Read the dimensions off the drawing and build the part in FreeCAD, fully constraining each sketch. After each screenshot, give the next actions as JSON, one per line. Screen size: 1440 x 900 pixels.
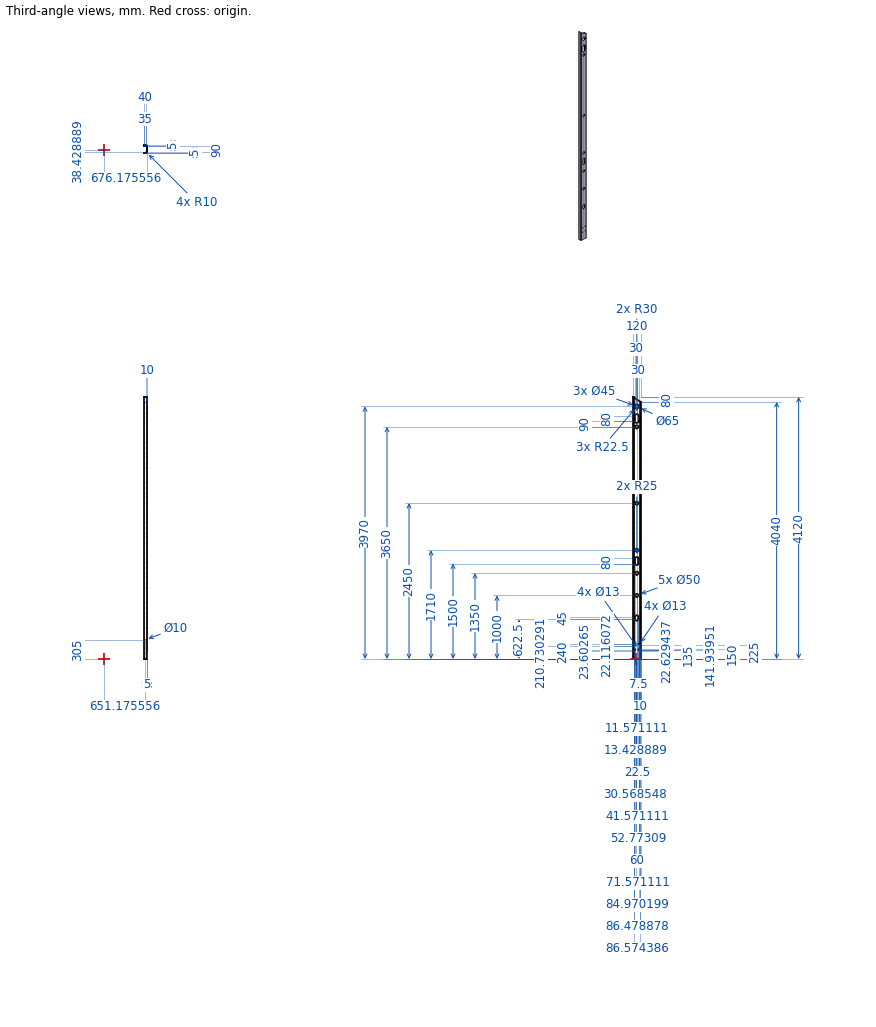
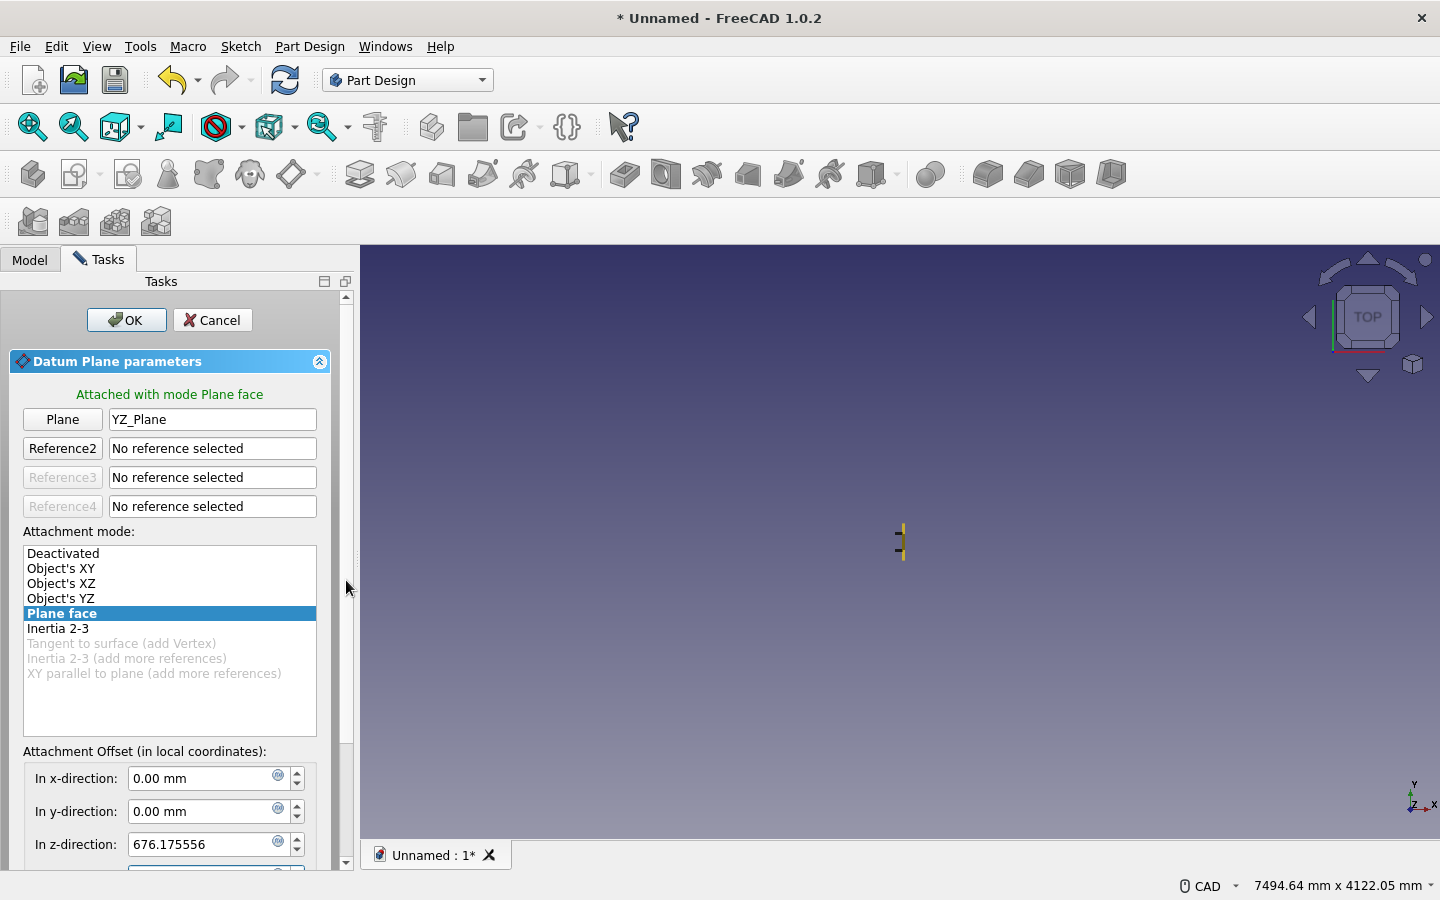
{"action": "left_click", "coordinate": [127, 320]}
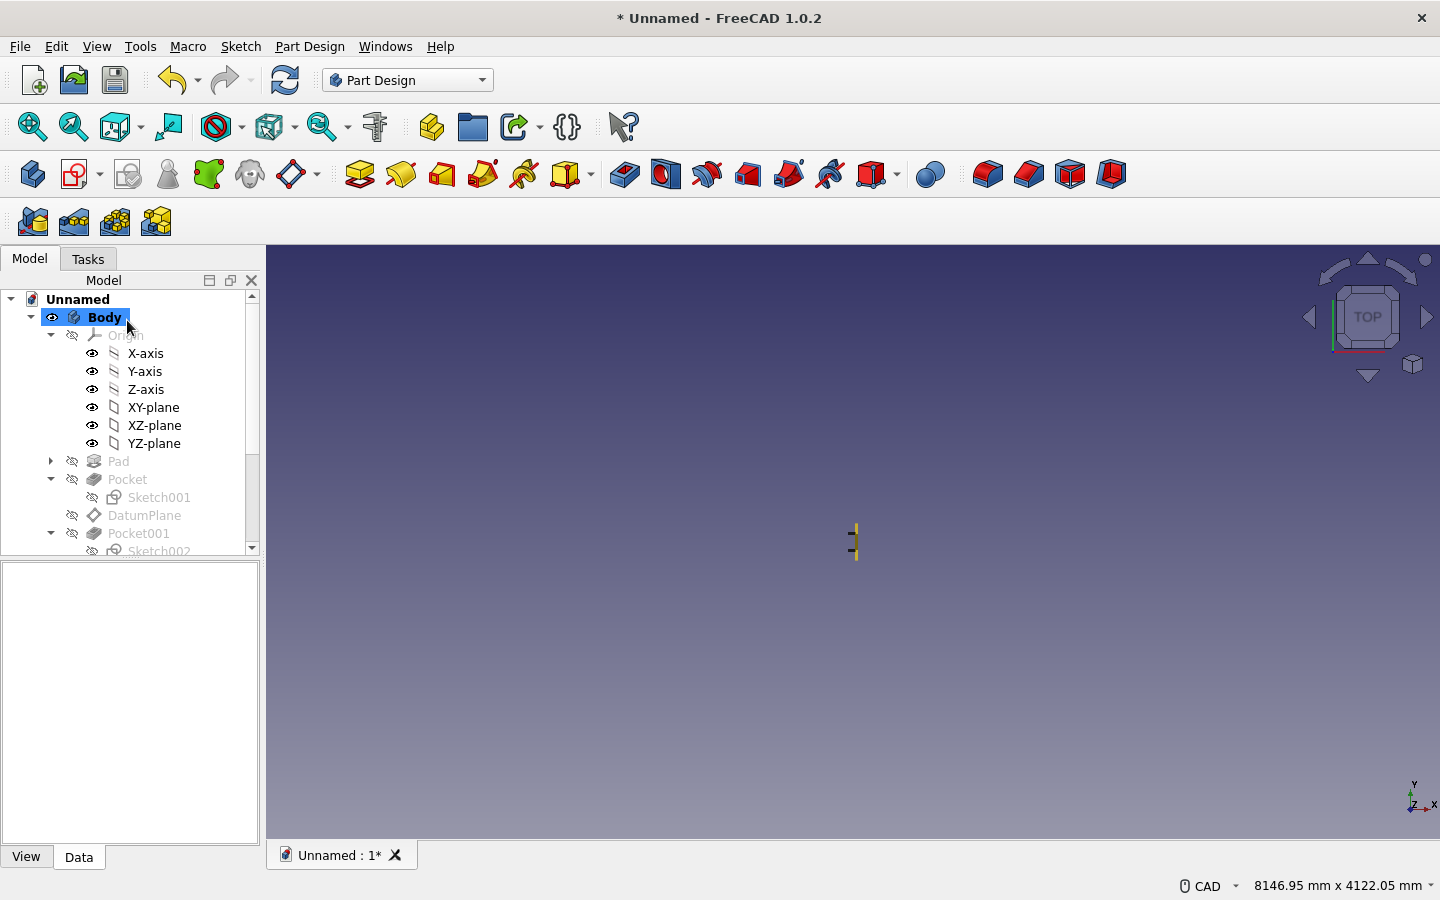
{"action": "scroll", "coordinate": [101, 421], "scroll_direction": "down", "scroll_amount": 3}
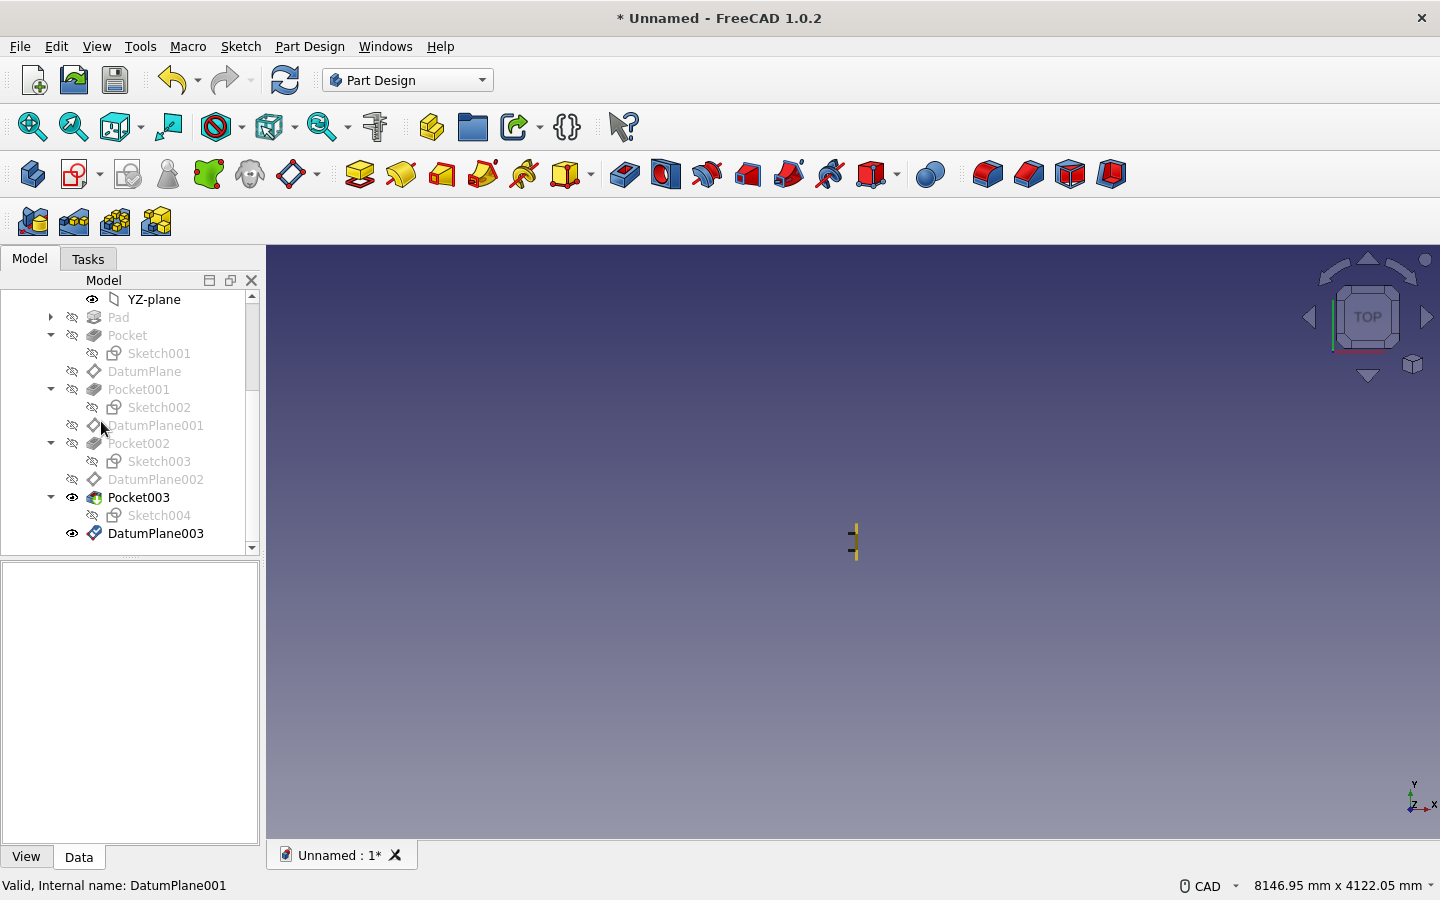
{"action": "left_click", "coordinate": [117, 533]}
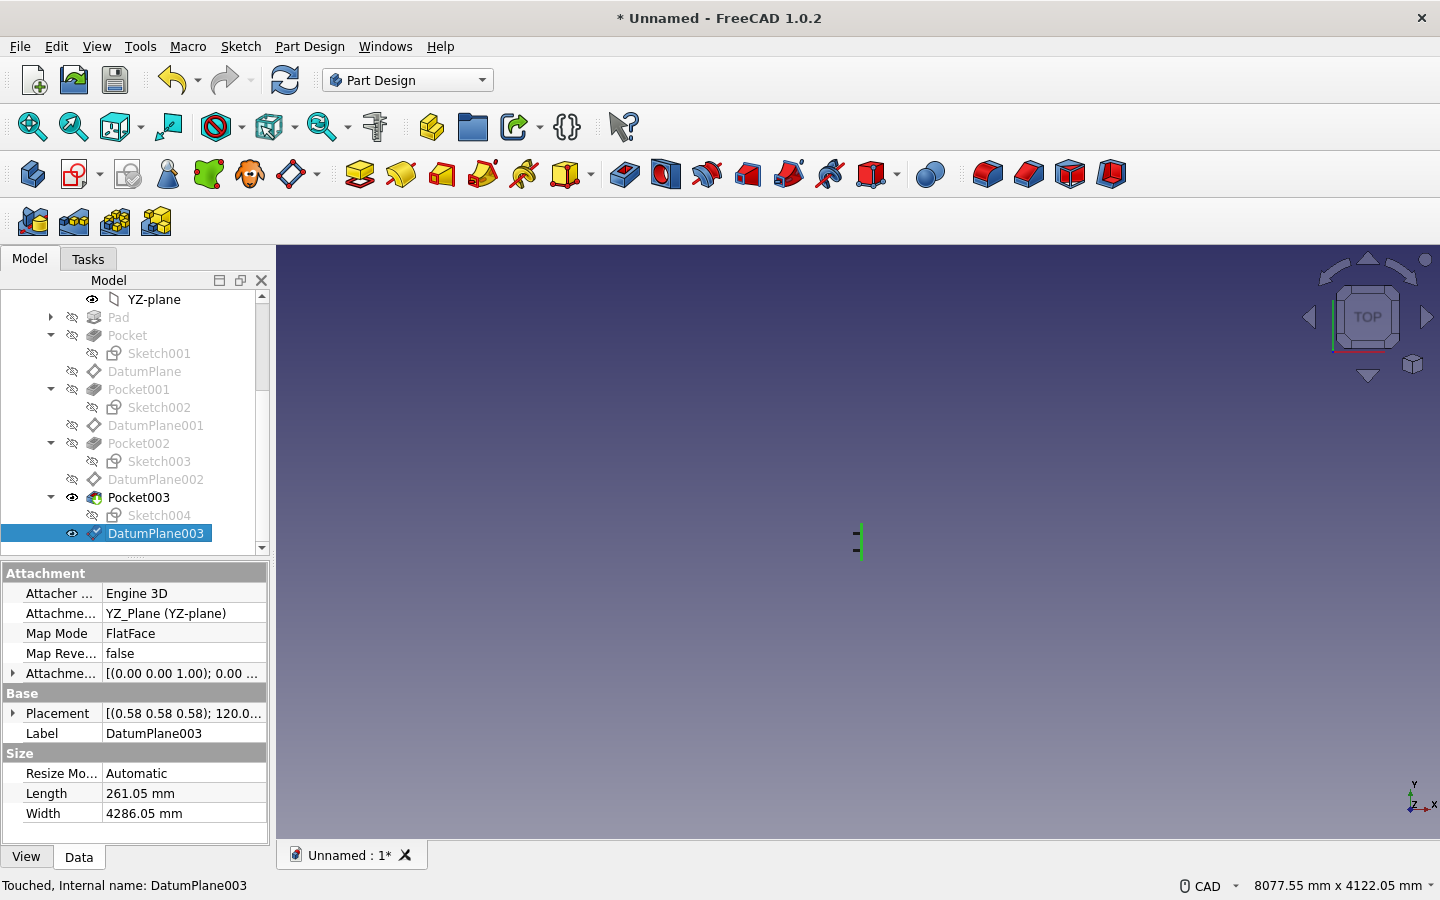
{"action": "left_click", "coordinate": [74, 174]}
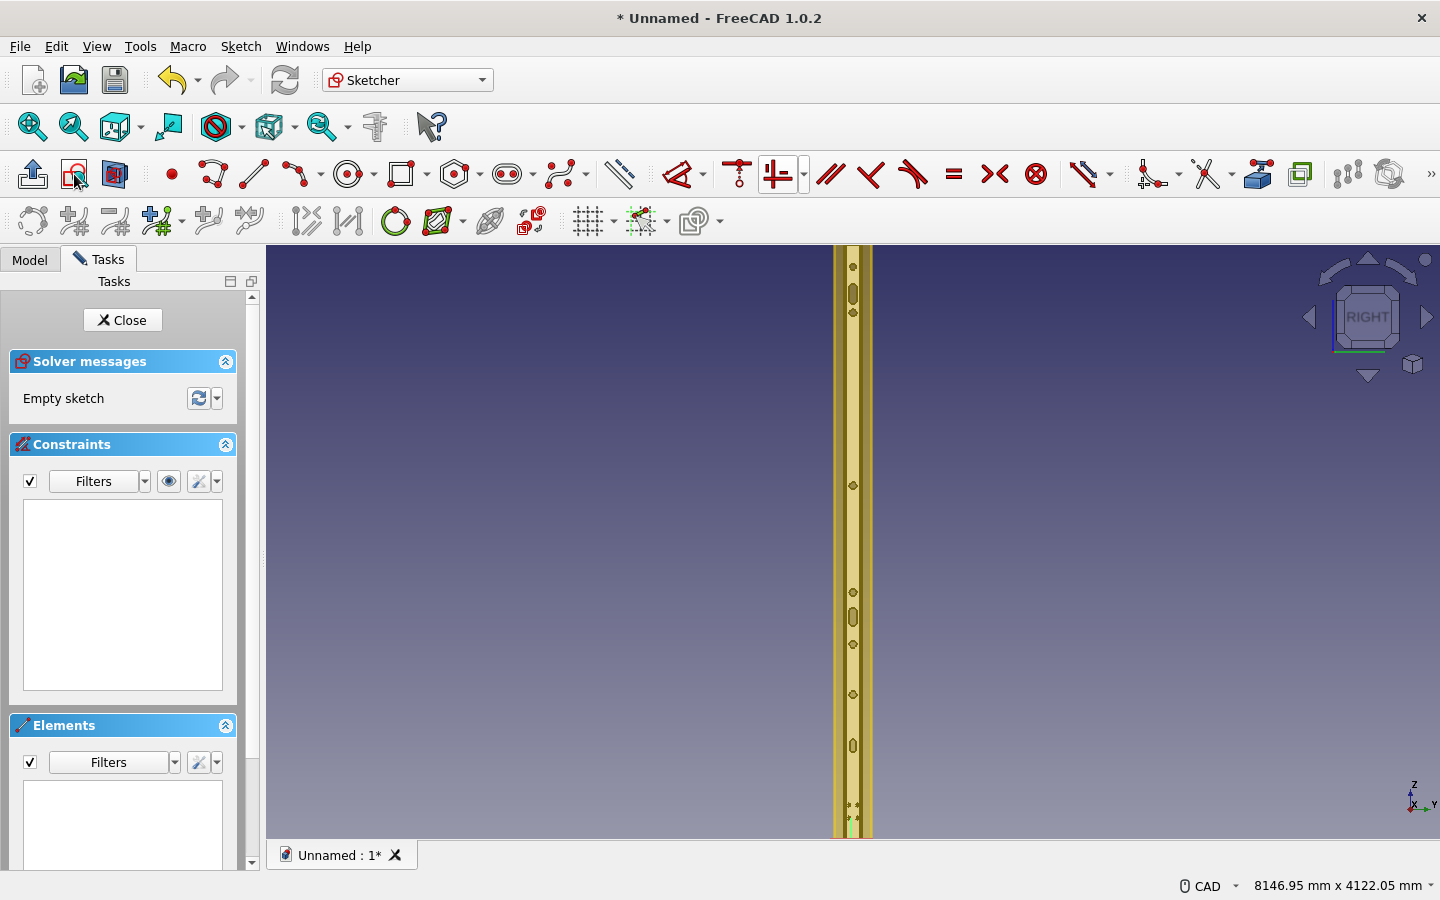
{"action": "scroll", "coordinate": [784, 542], "scroll_direction": "down", "scroll_amount": 5}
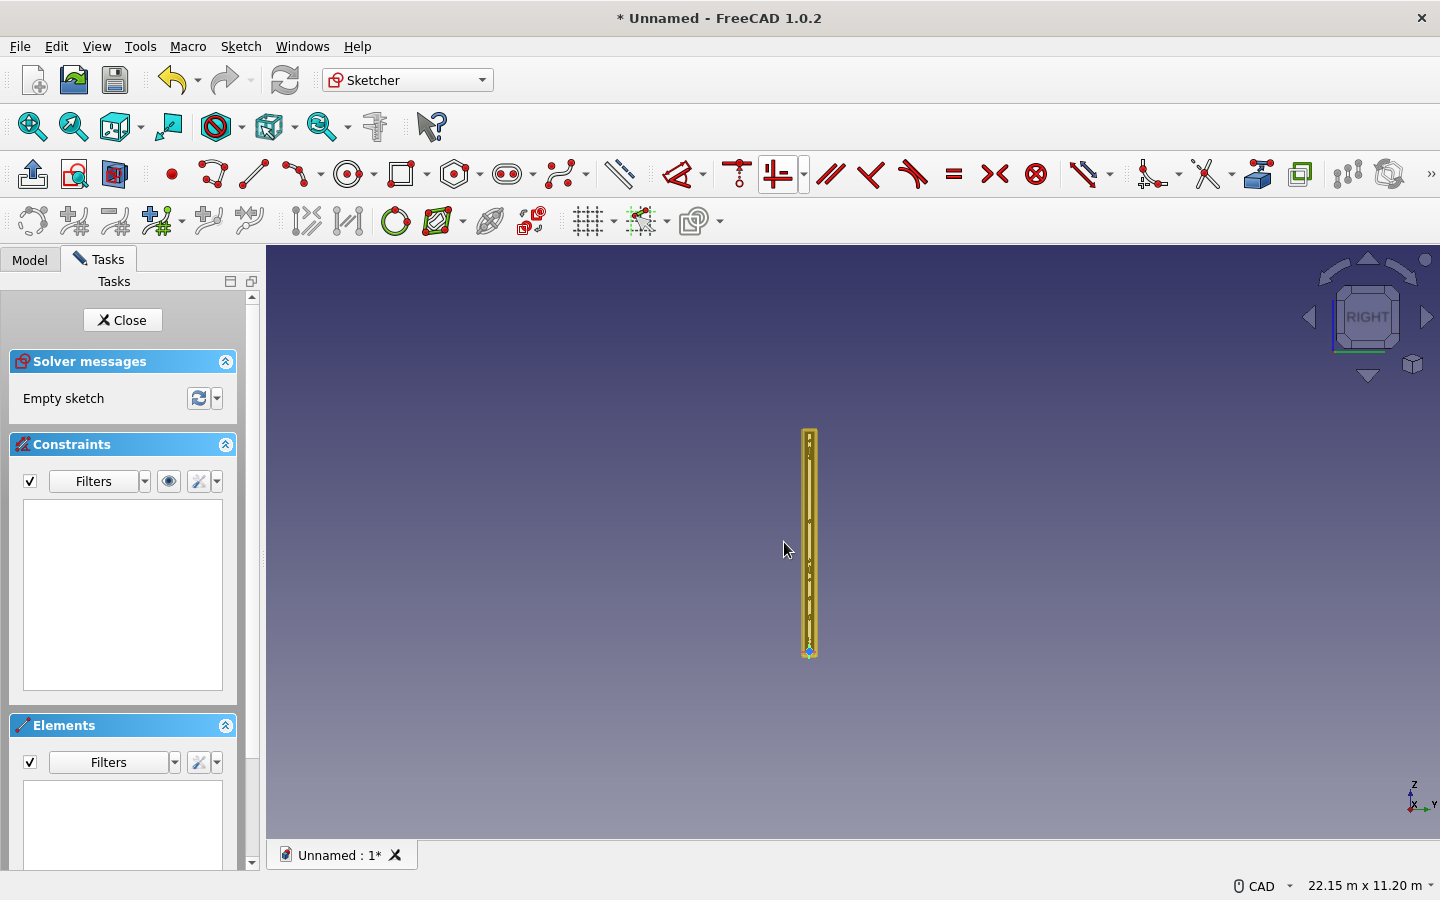
{"action": "scroll", "coordinate": [811, 651], "scroll_direction": "up", "scroll_amount": 15}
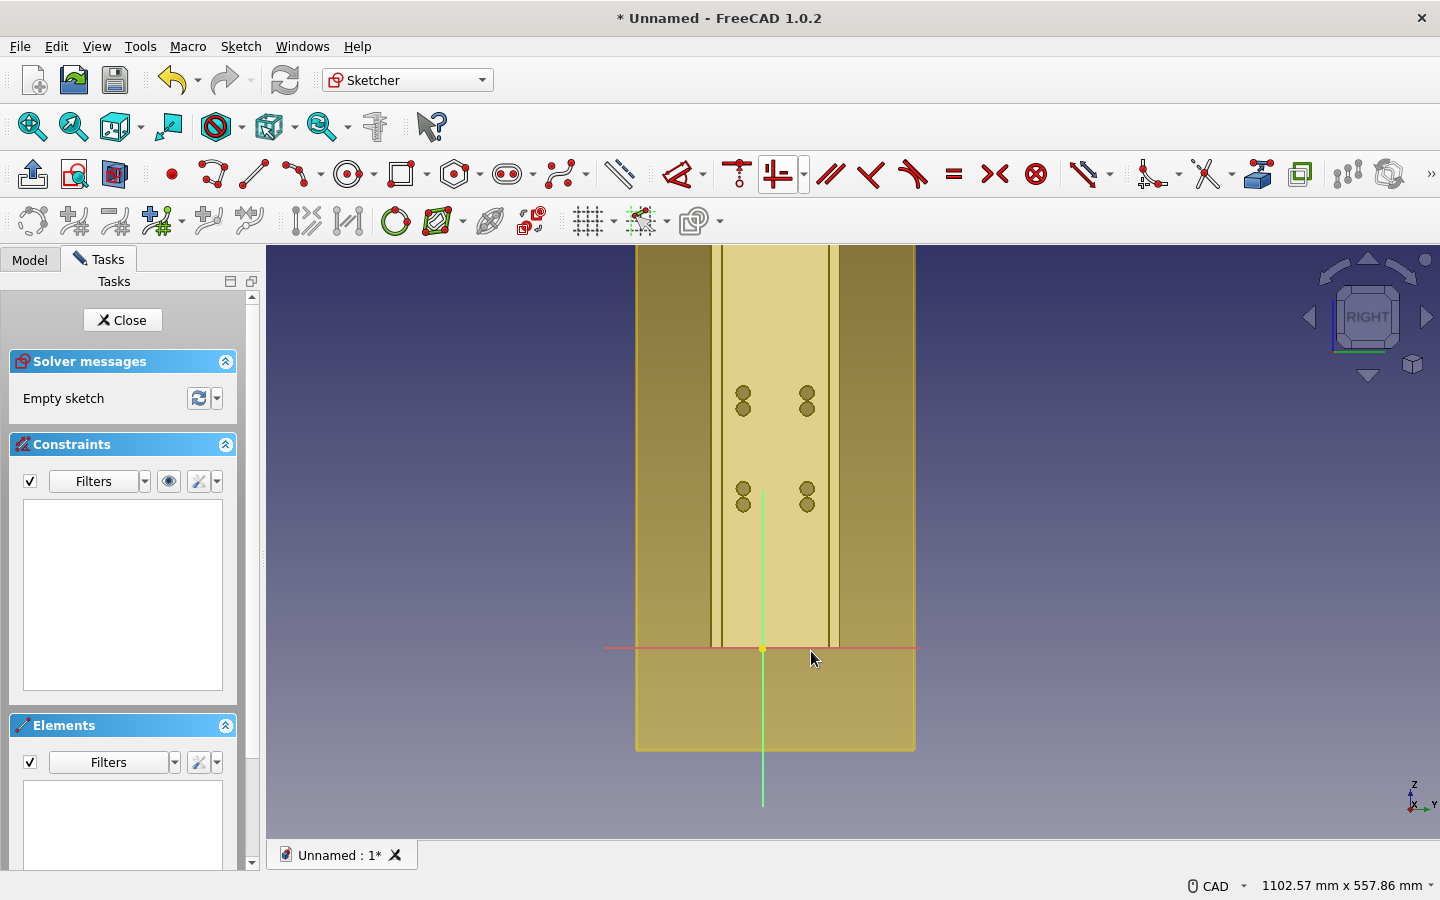
{"action": "scroll", "coordinate": [758, 489], "scroll_direction": "up", "scroll_amount": 2}